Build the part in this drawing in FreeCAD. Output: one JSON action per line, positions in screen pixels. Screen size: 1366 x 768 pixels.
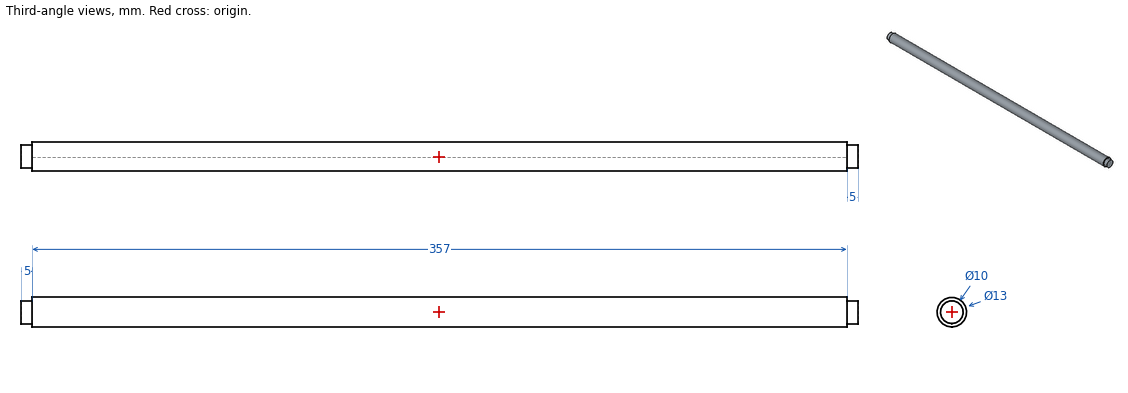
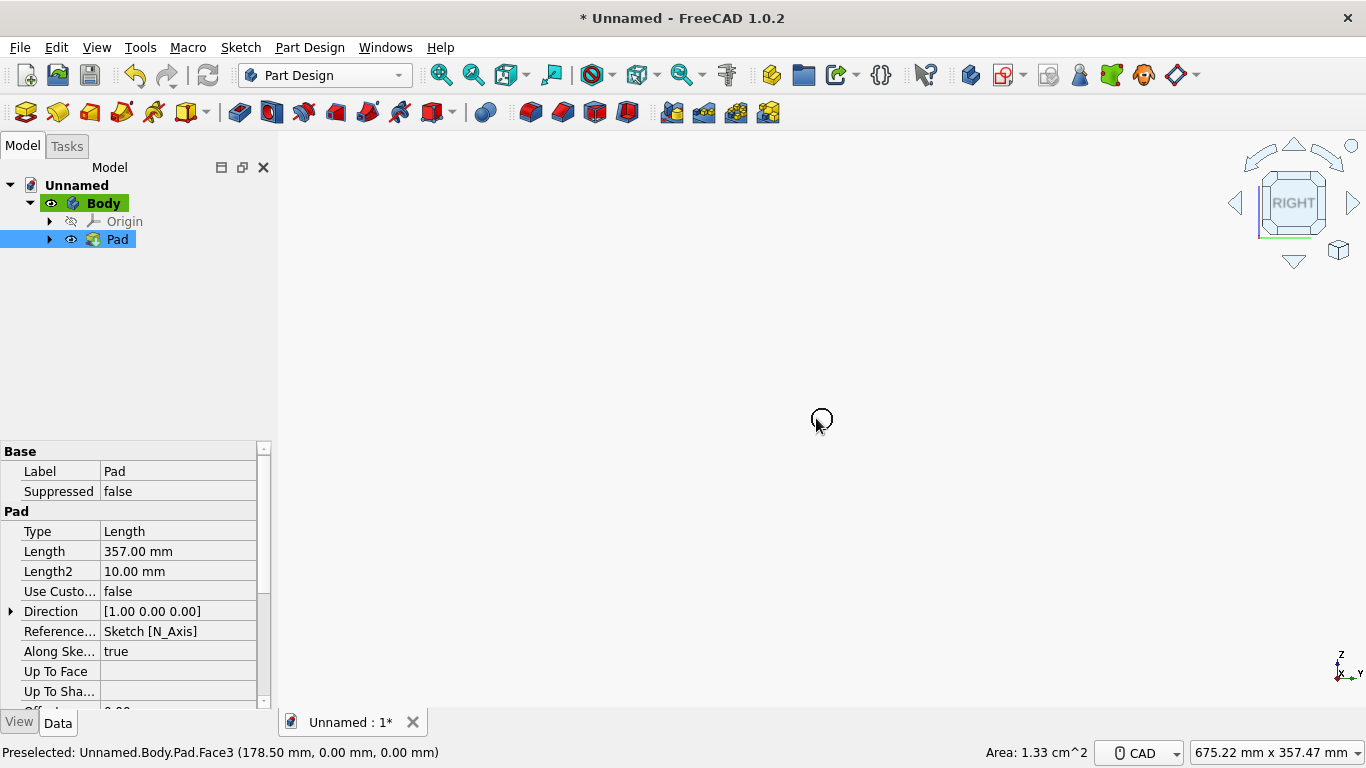
{"action": "left_click", "coordinate": [1004, 76]}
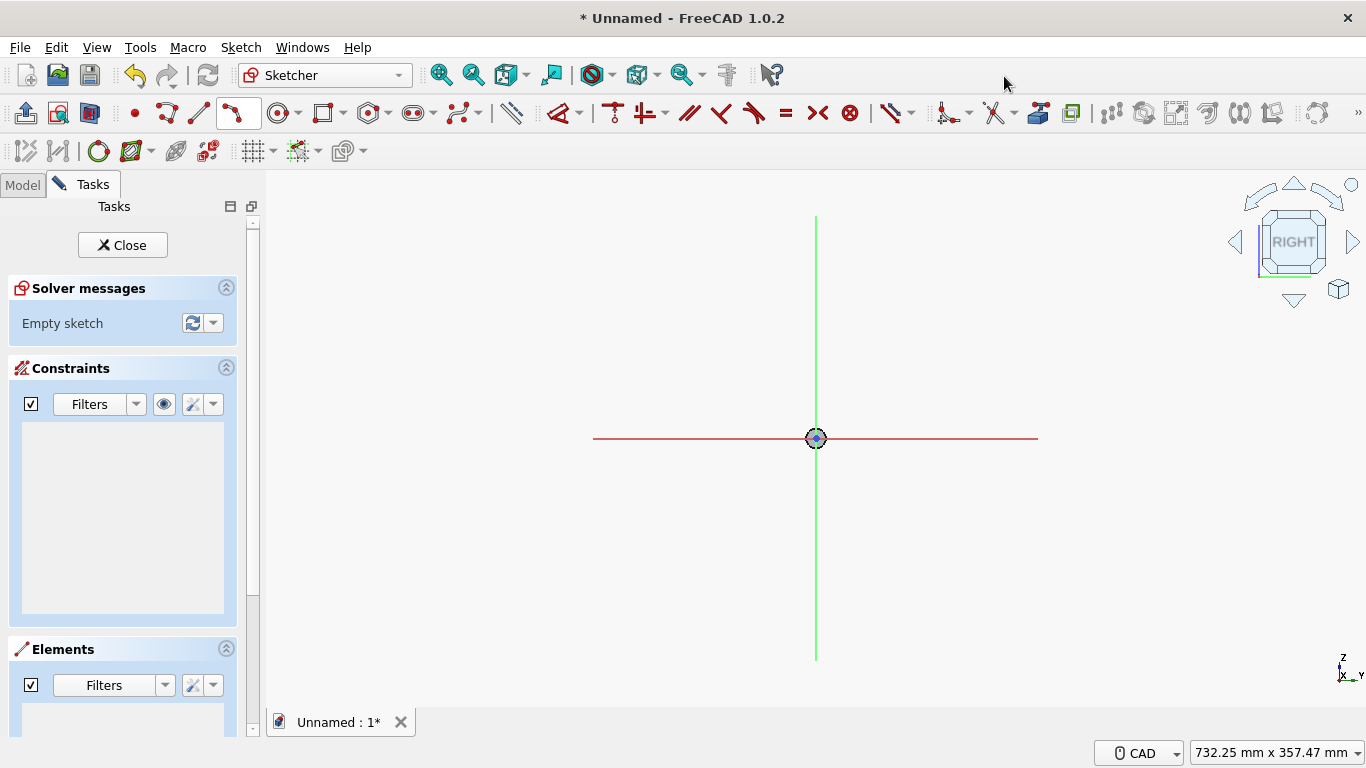
{"action": "scroll", "coordinate": [820, 438], "scroll_direction": "up", "scroll_amount": 15}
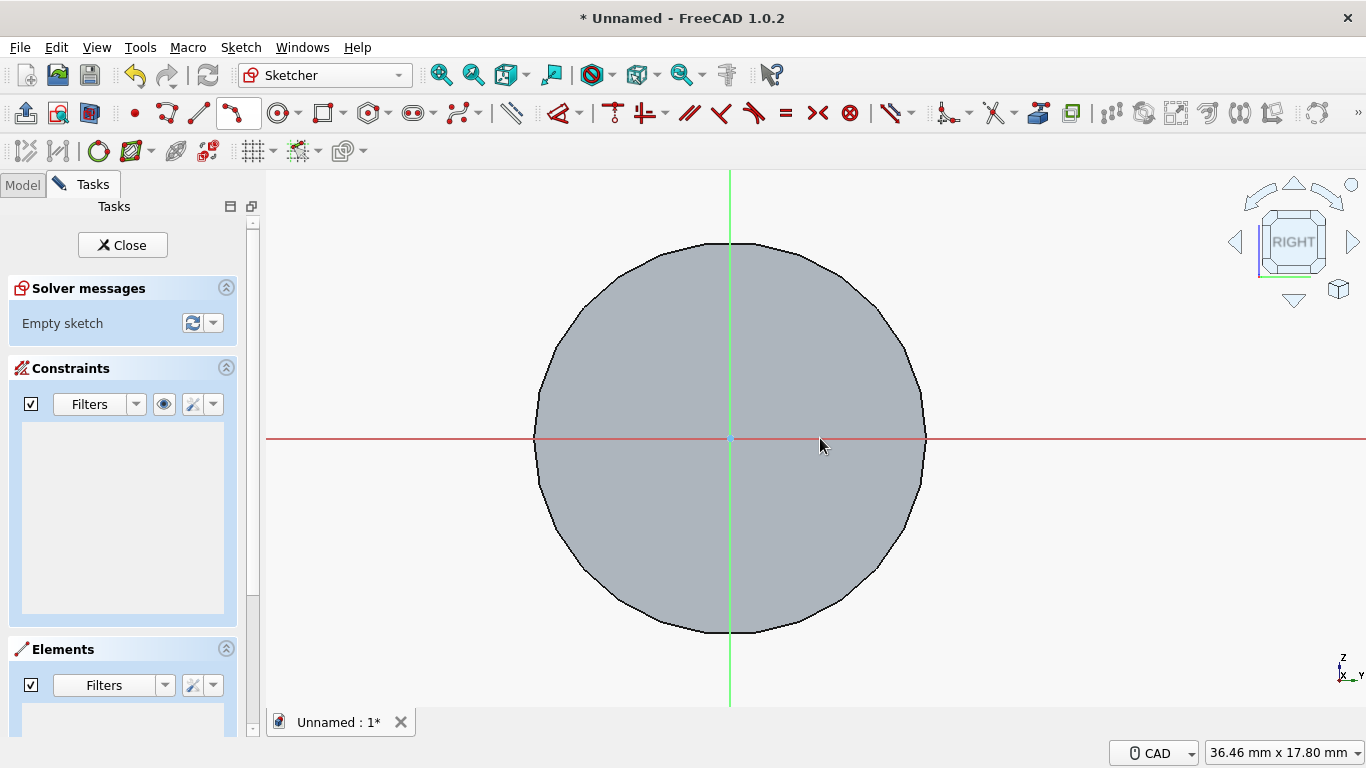
{"action": "left_click", "coordinate": [278, 114]}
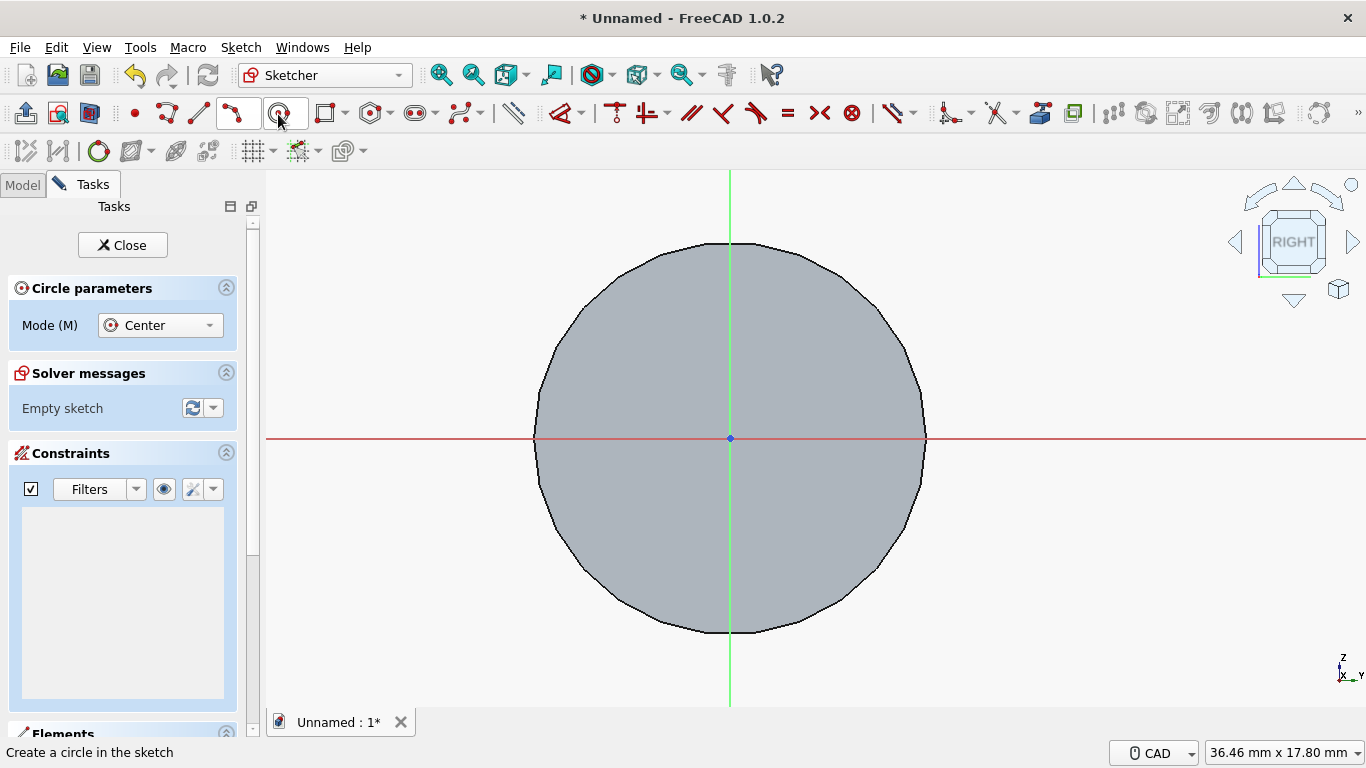
{"action": "left_click", "coordinate": [730, 438]}
{"action": "left_click", "coordinate": [837, 332]}
{"action": "key", "text": "Escape"}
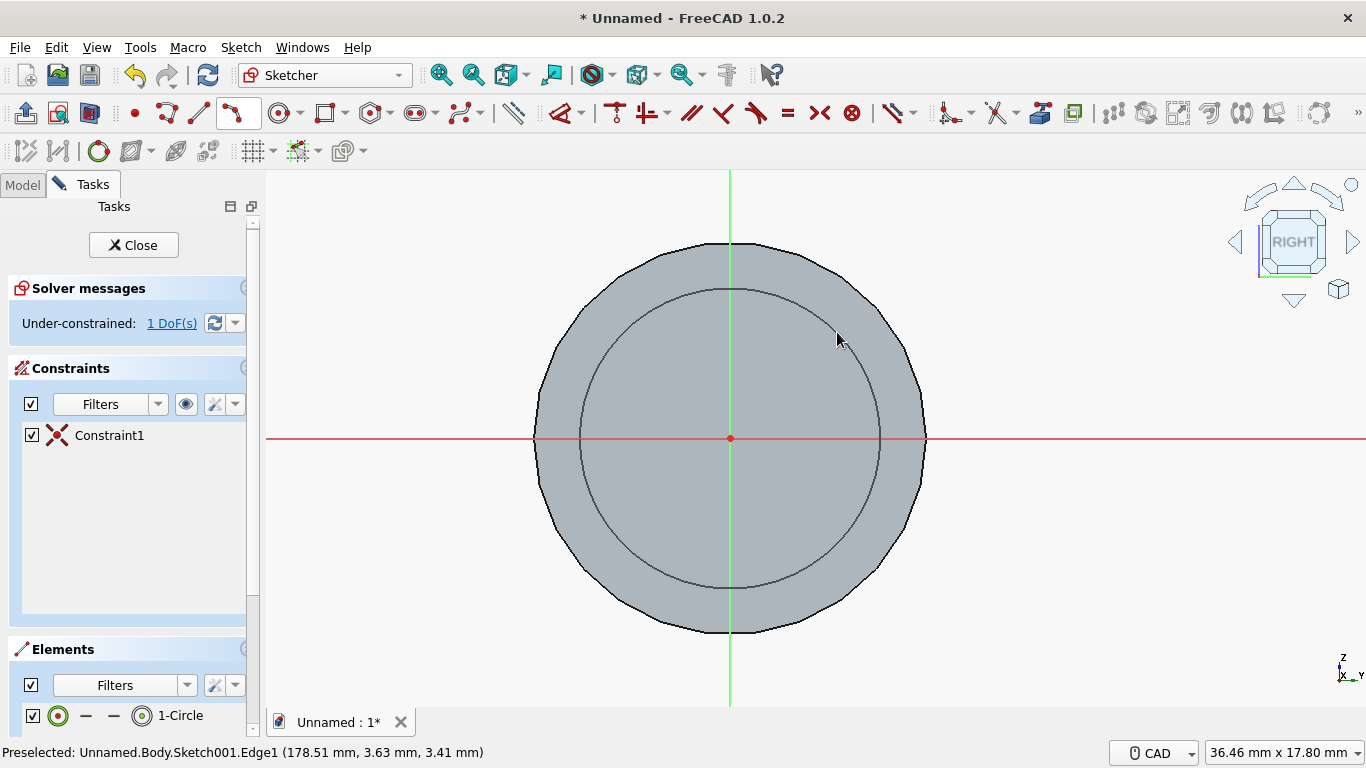
{"action": "left_click", "coordinate": [836, 332]}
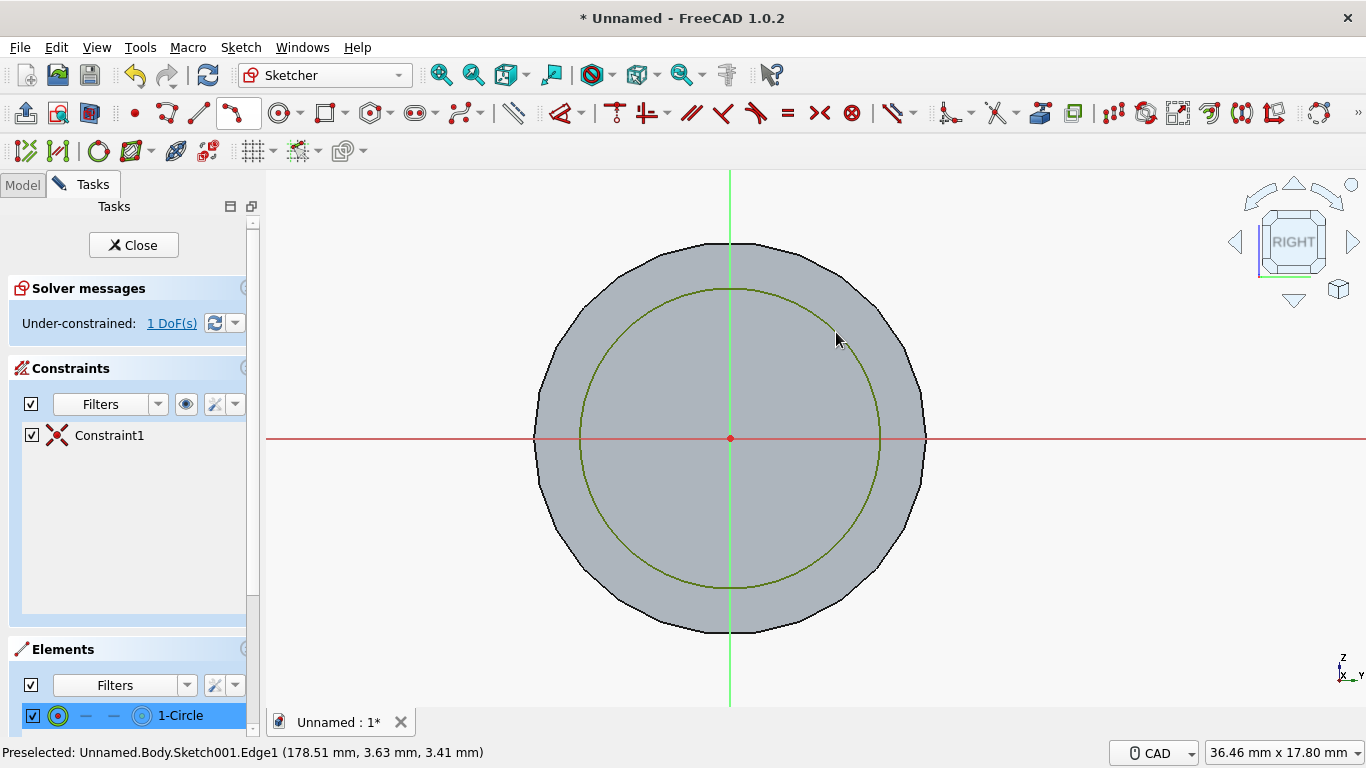
{"action": "left_click", "coordinate": [584, 114]}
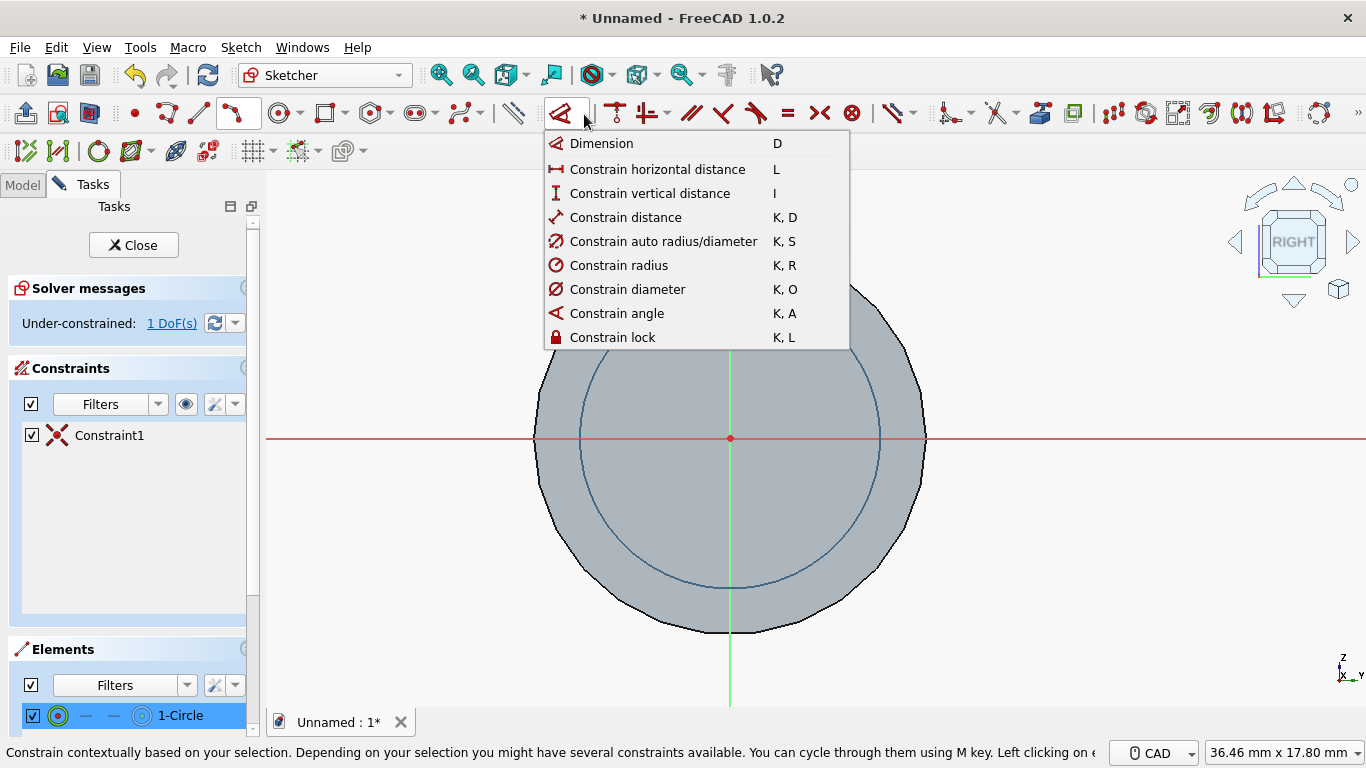
{"action": "left_click", "coordinate": [697, 289]}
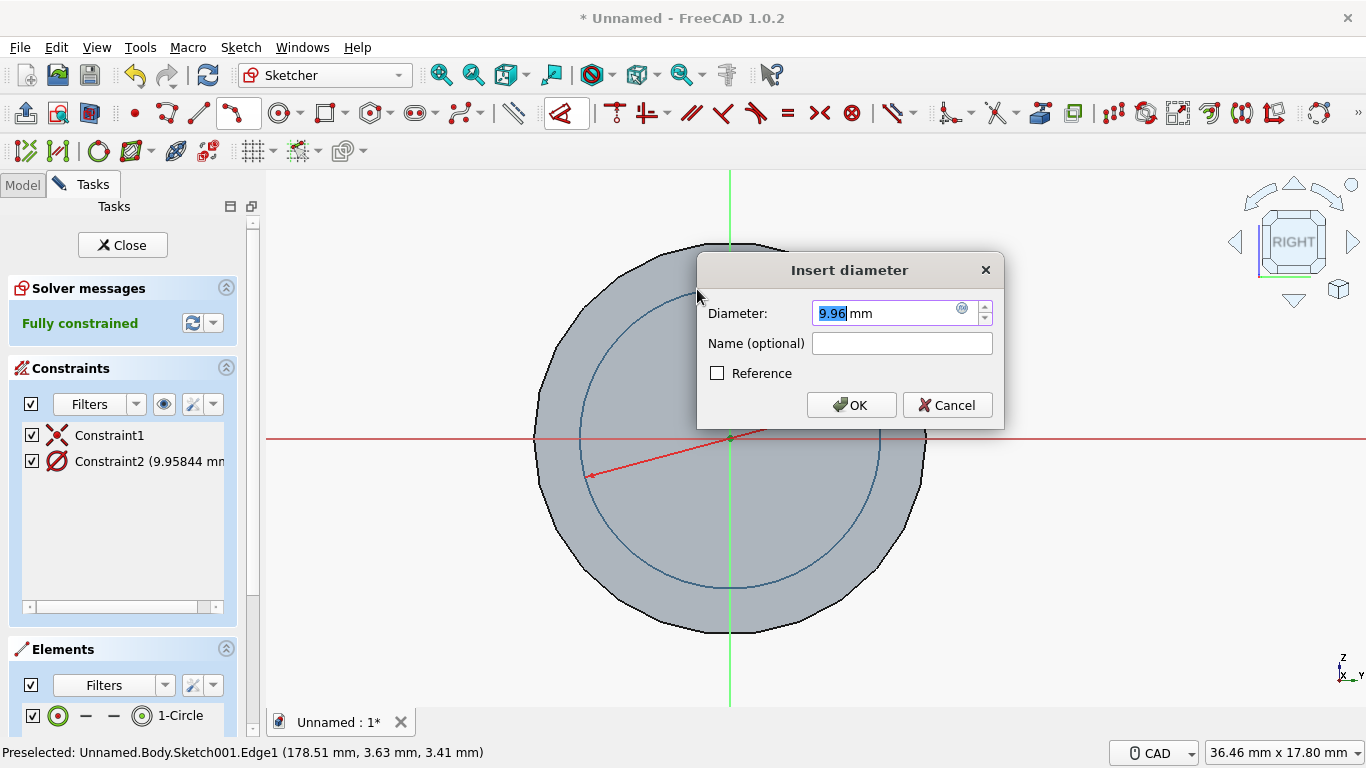
{"action": "type", "text": "10"}
{"action": "key", "text": "Return"}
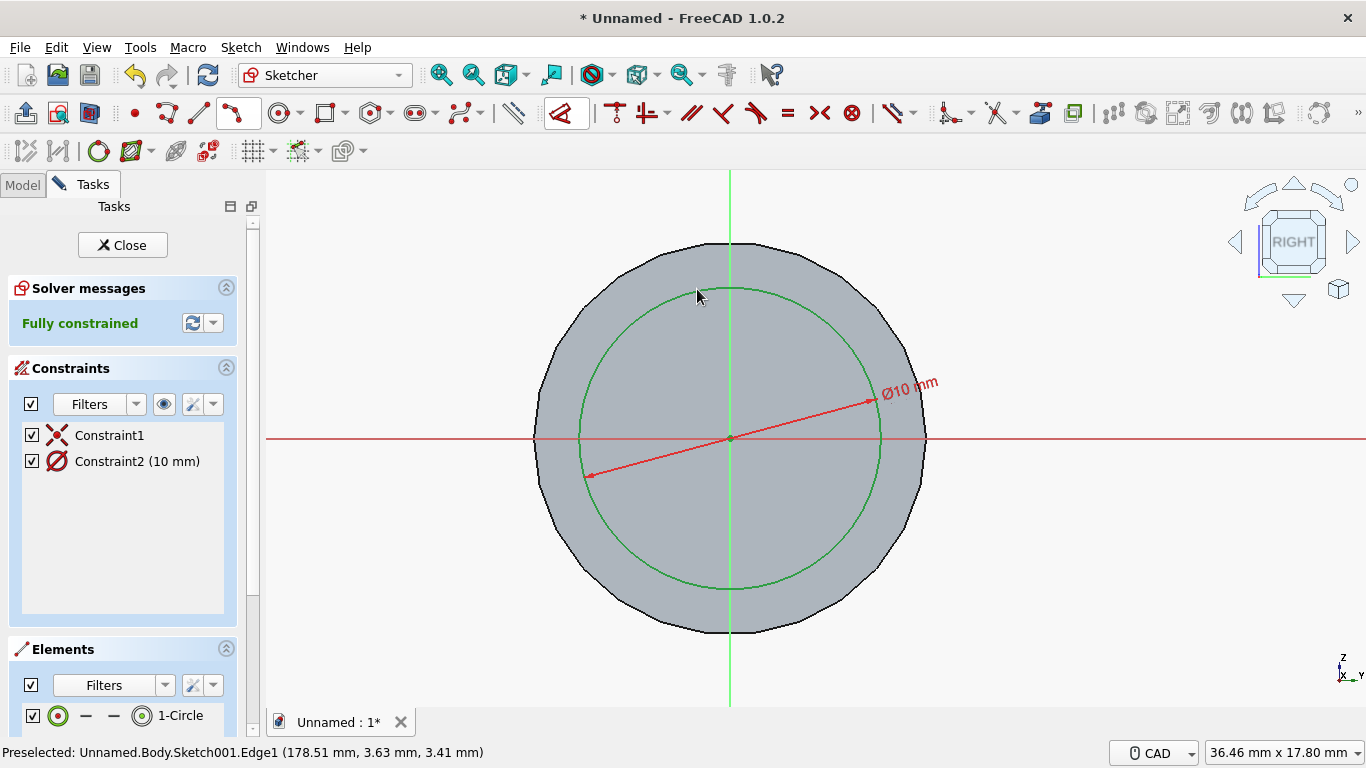
{"action": "left_click", "coordinate": [123, 245]}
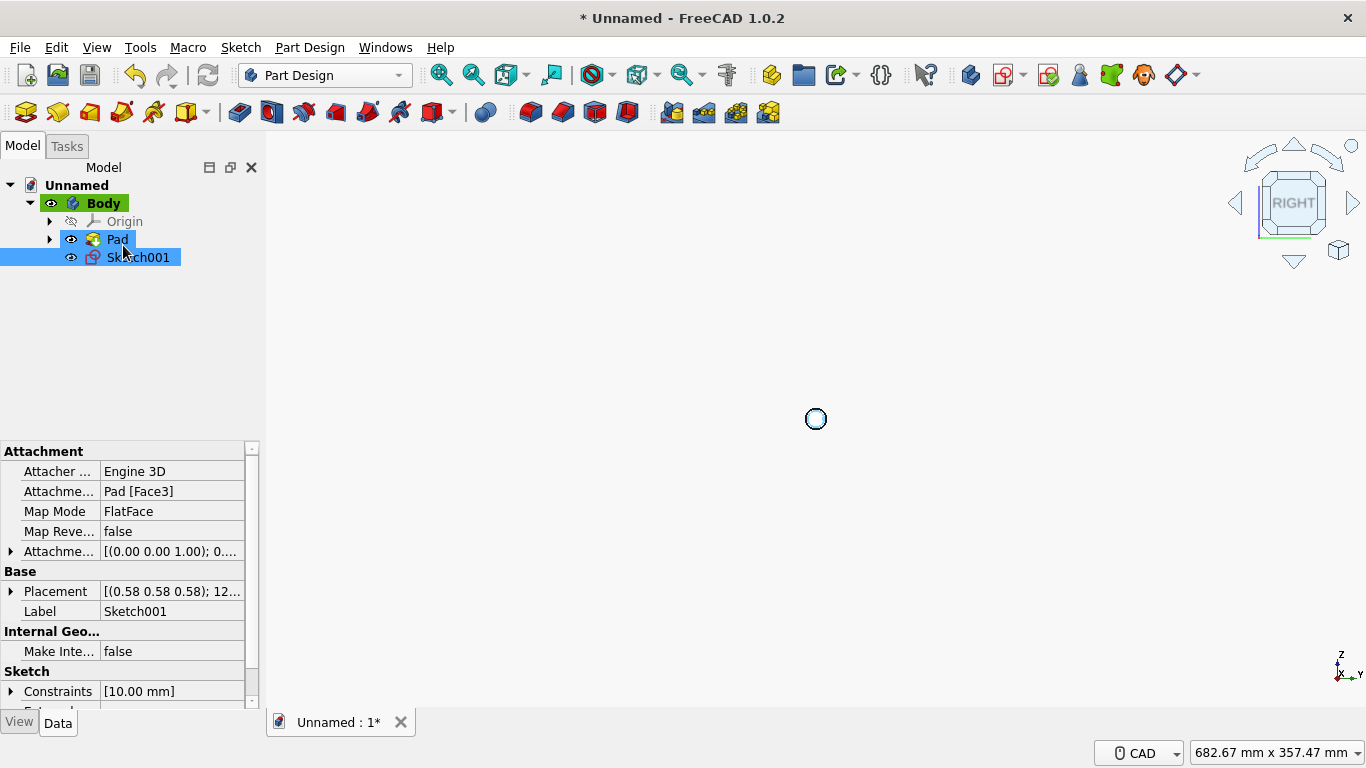
{"action": "left_click", "coordinate": [26, 112]}